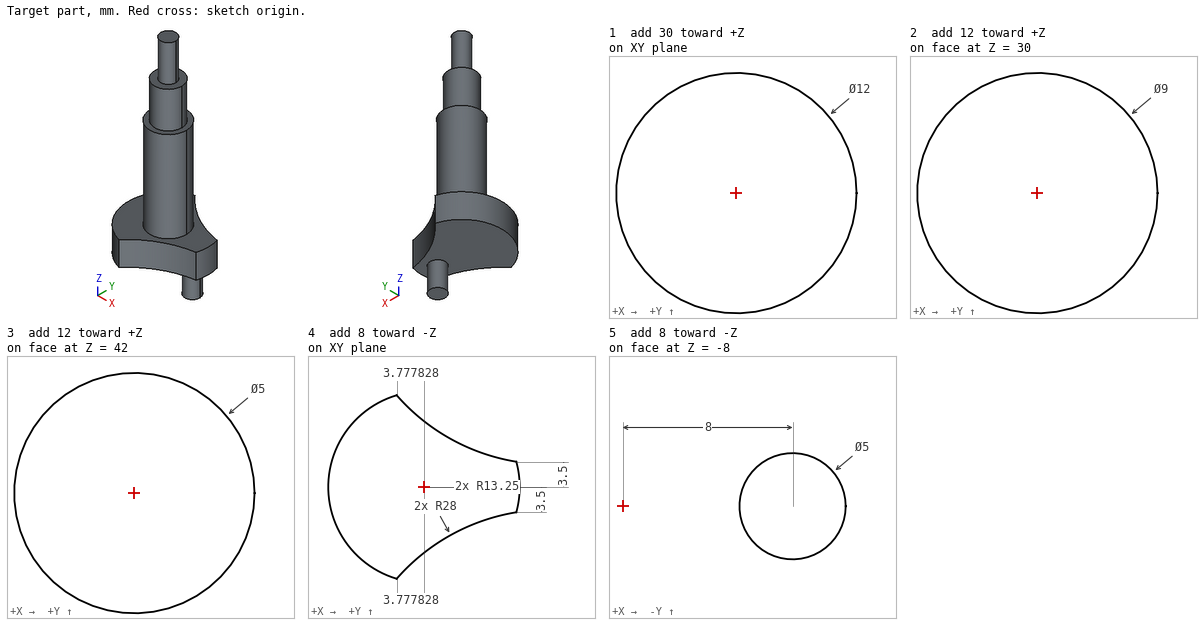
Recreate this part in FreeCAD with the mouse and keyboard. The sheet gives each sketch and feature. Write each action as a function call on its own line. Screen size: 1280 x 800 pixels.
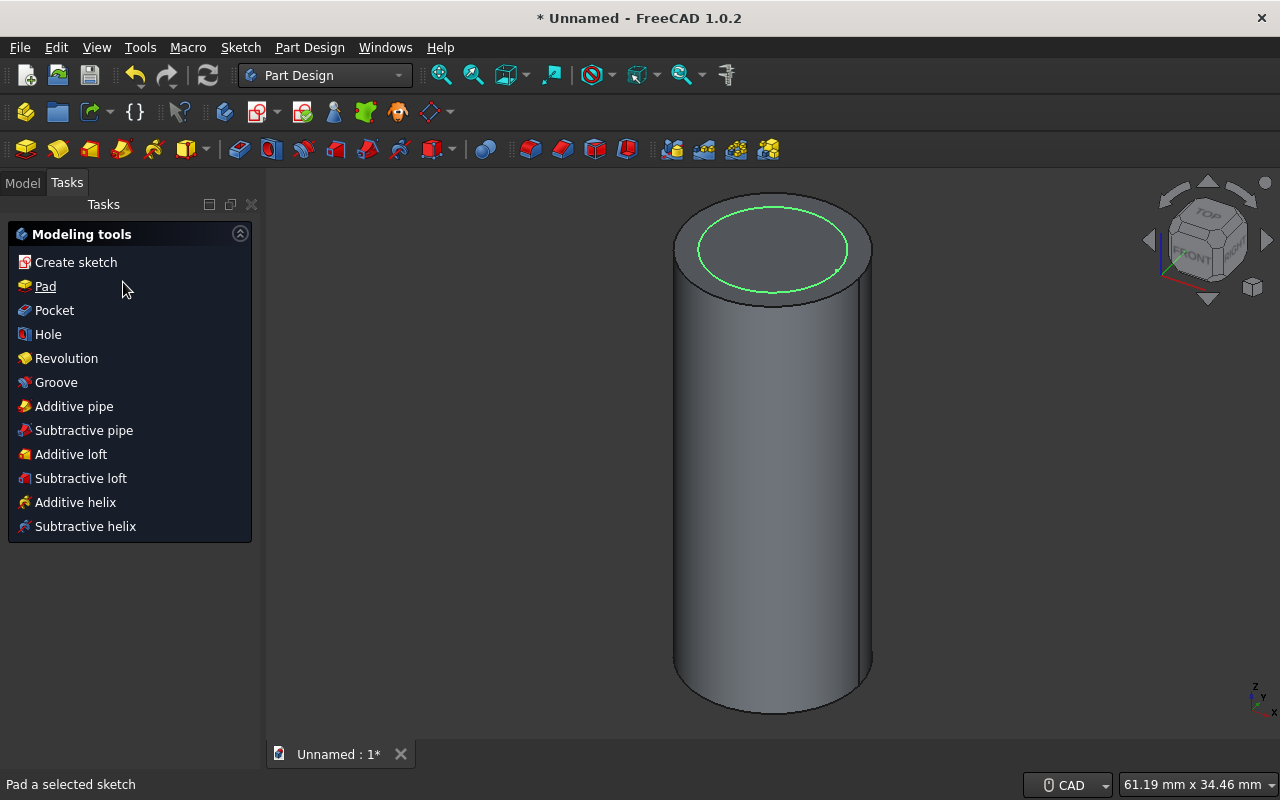
click(26, 150)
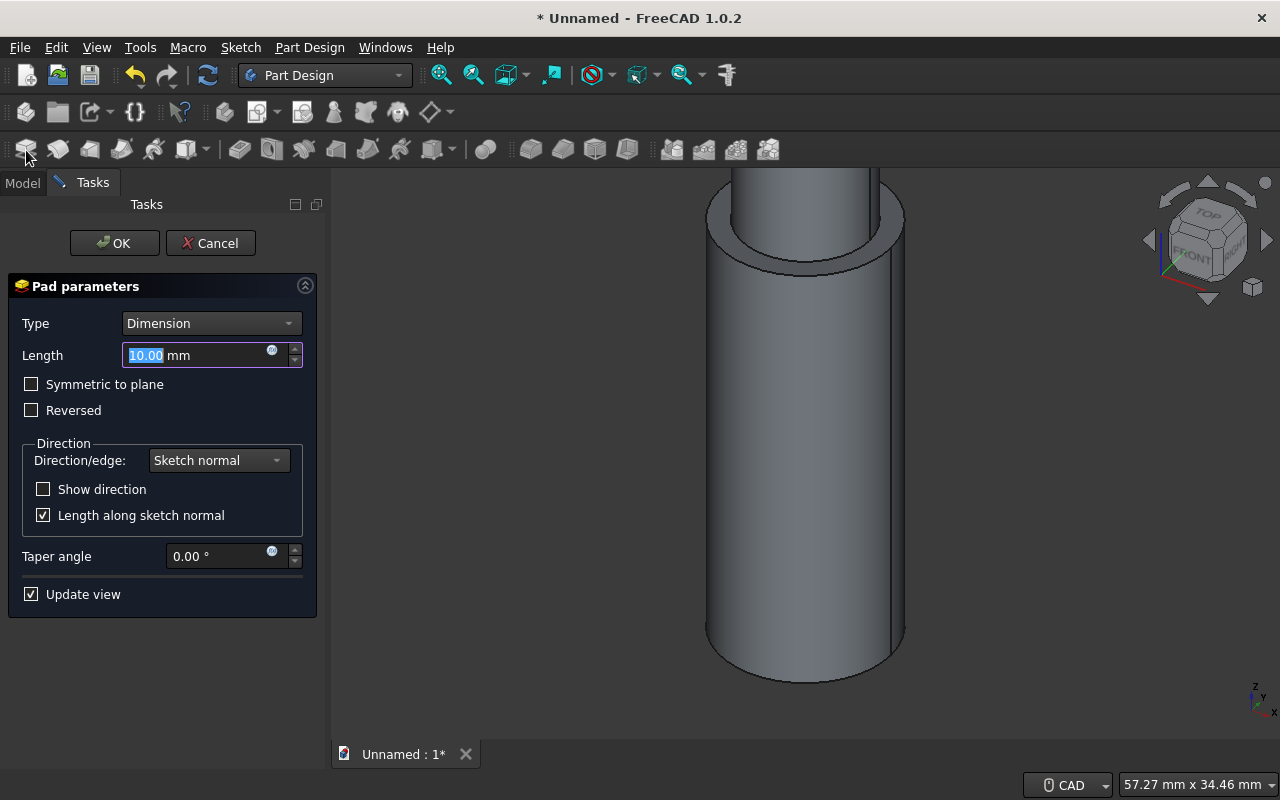
text(12)
key(Tab)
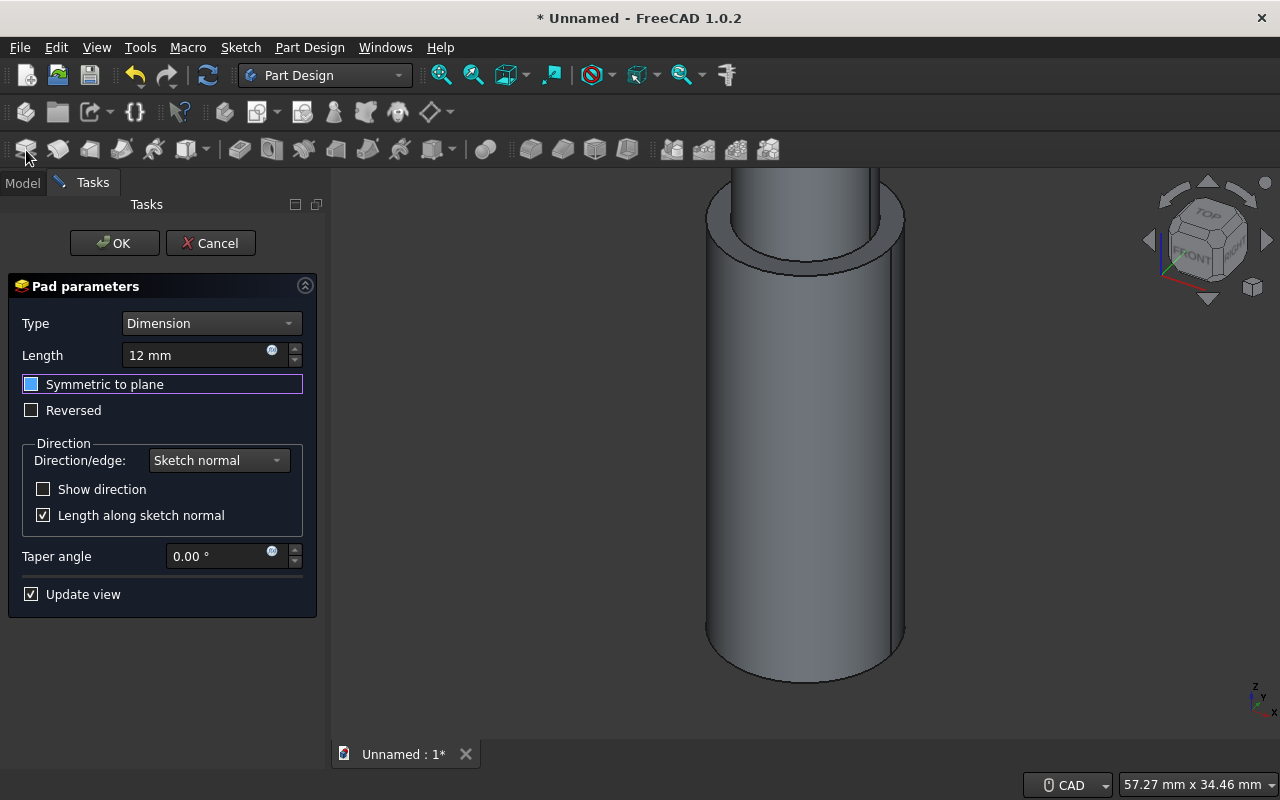
click(115, 243)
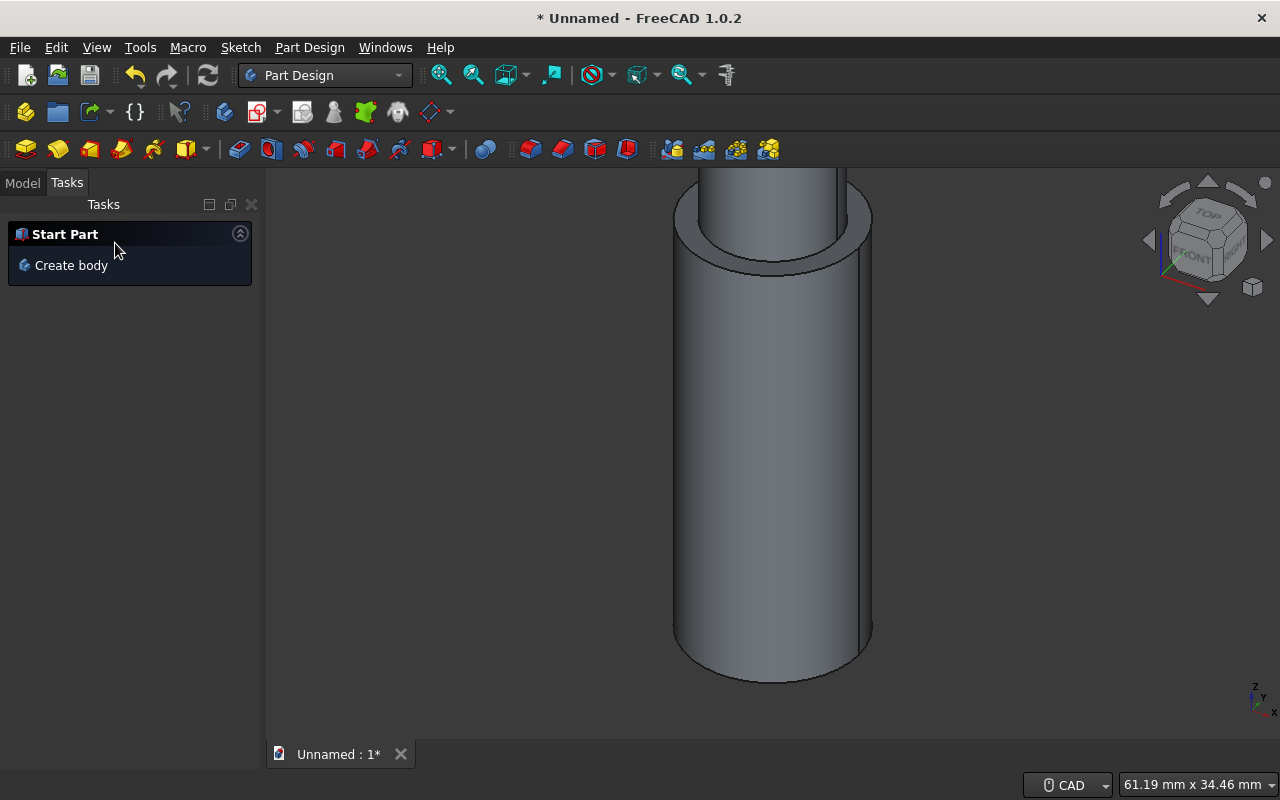
click(442, 76)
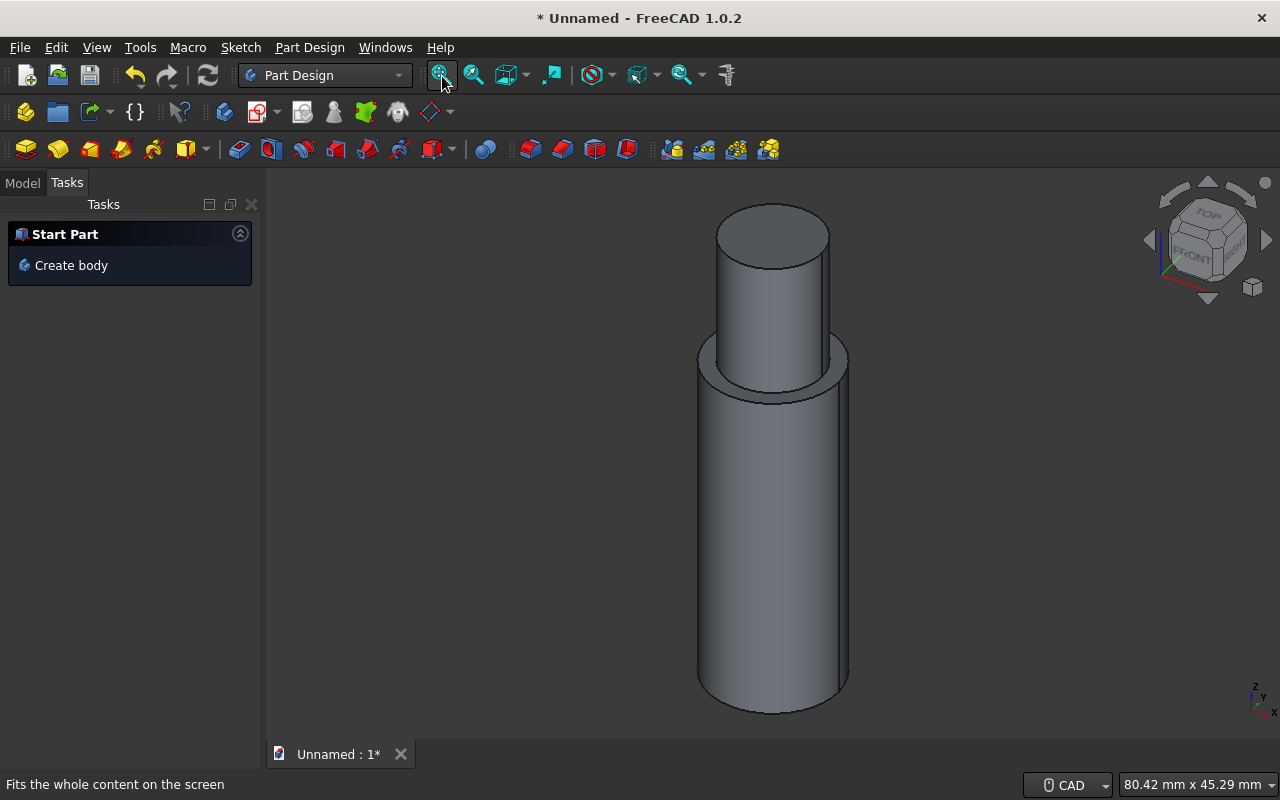
click(773, 236)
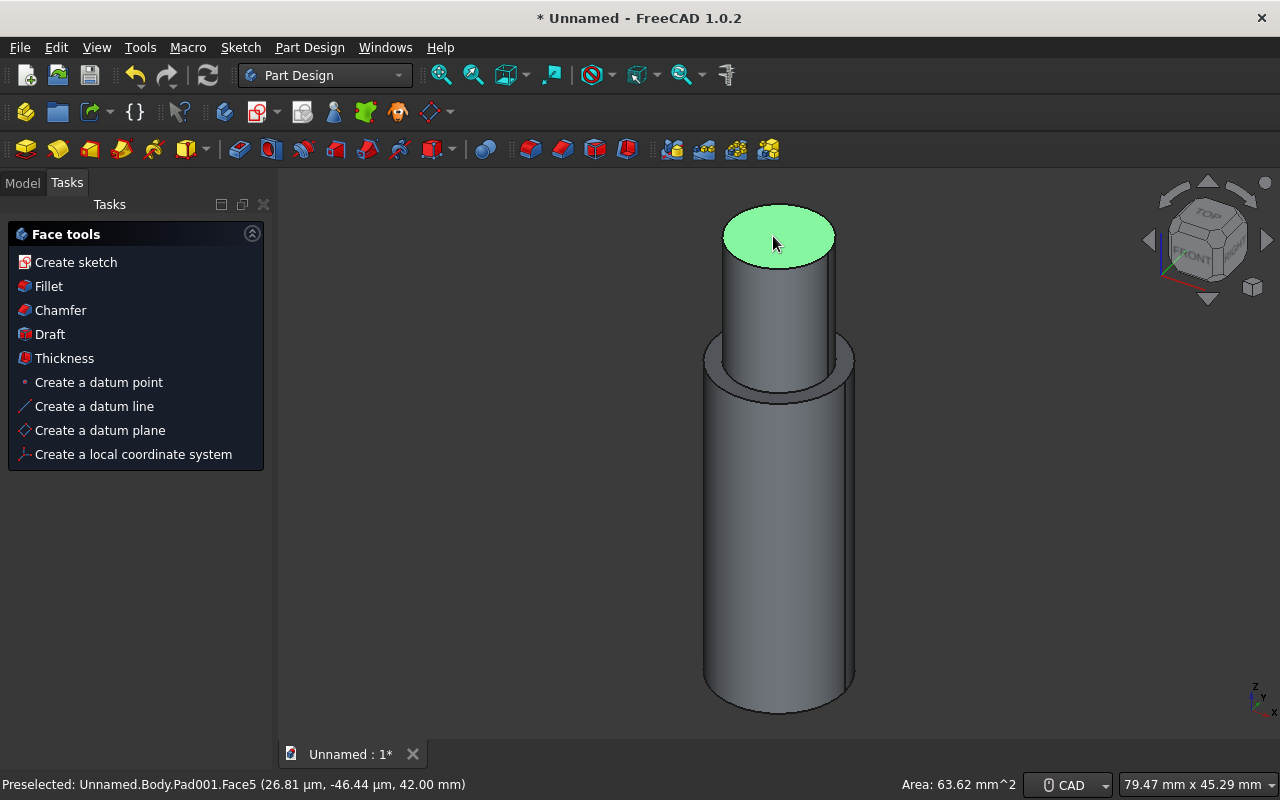
click(258, 112)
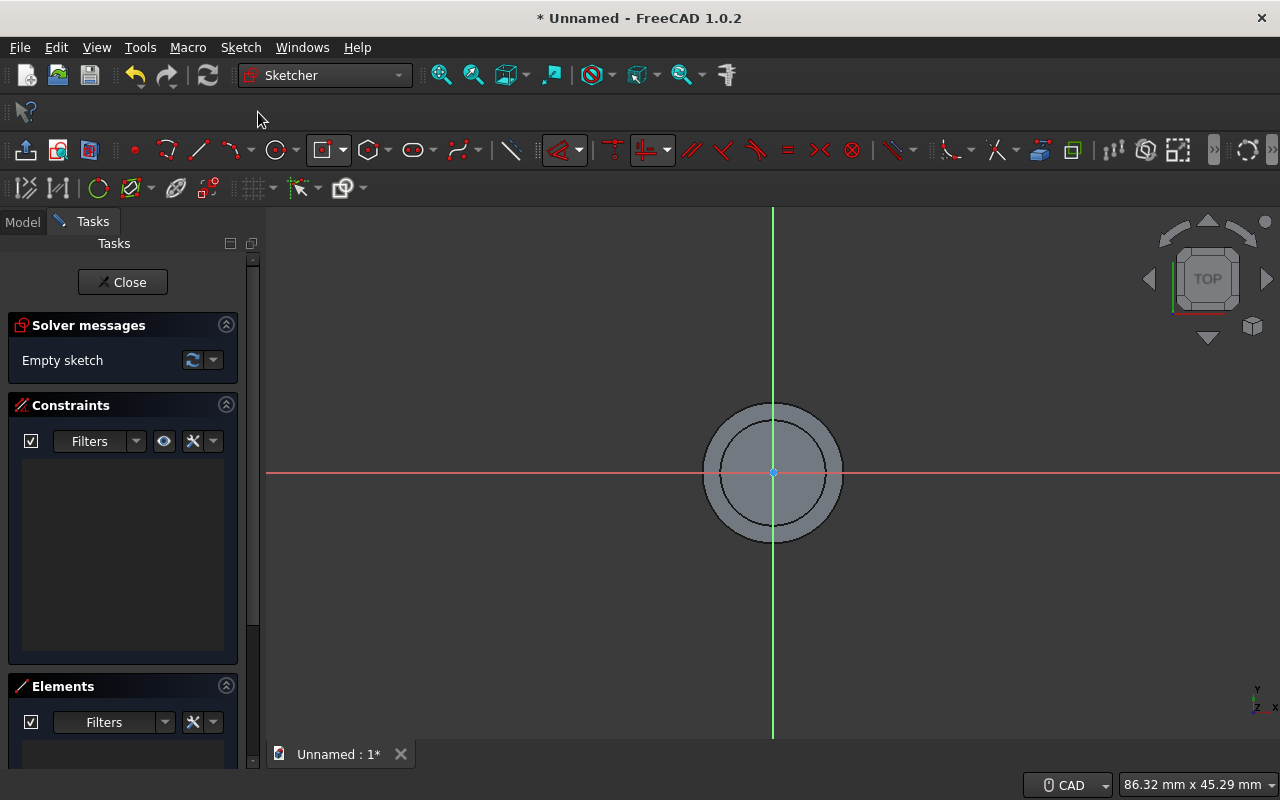
scroll(787, 473, up, 9)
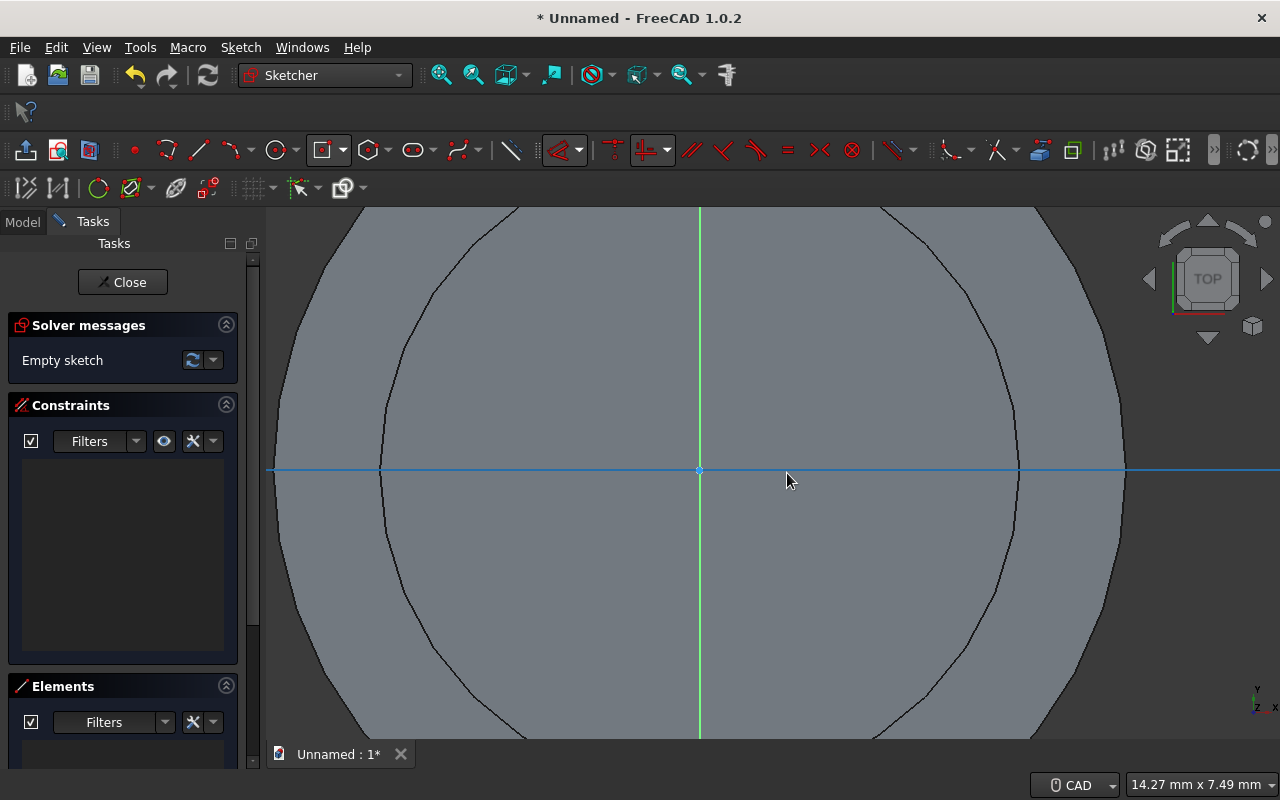
click(276, 150)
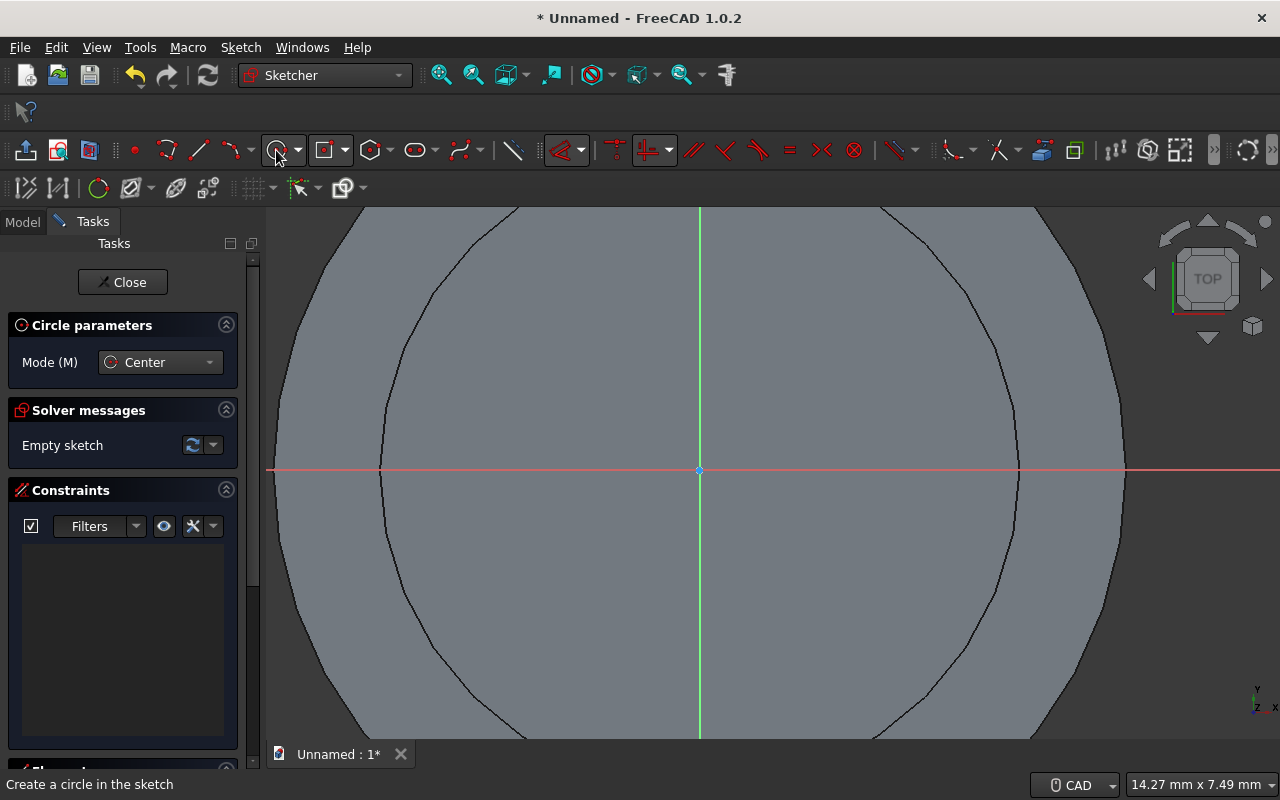
click(700, 470)
move(825, 345)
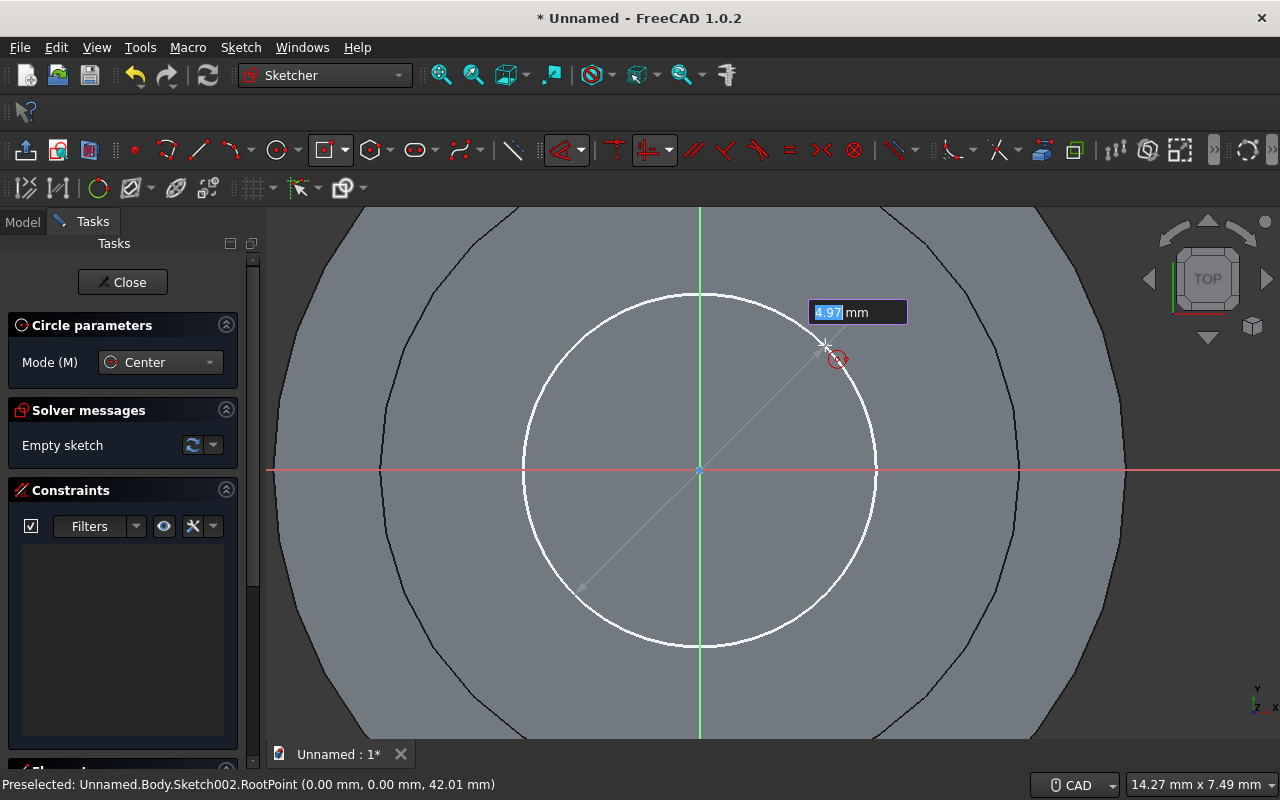
text(5)
key(Return)
key(Escape)